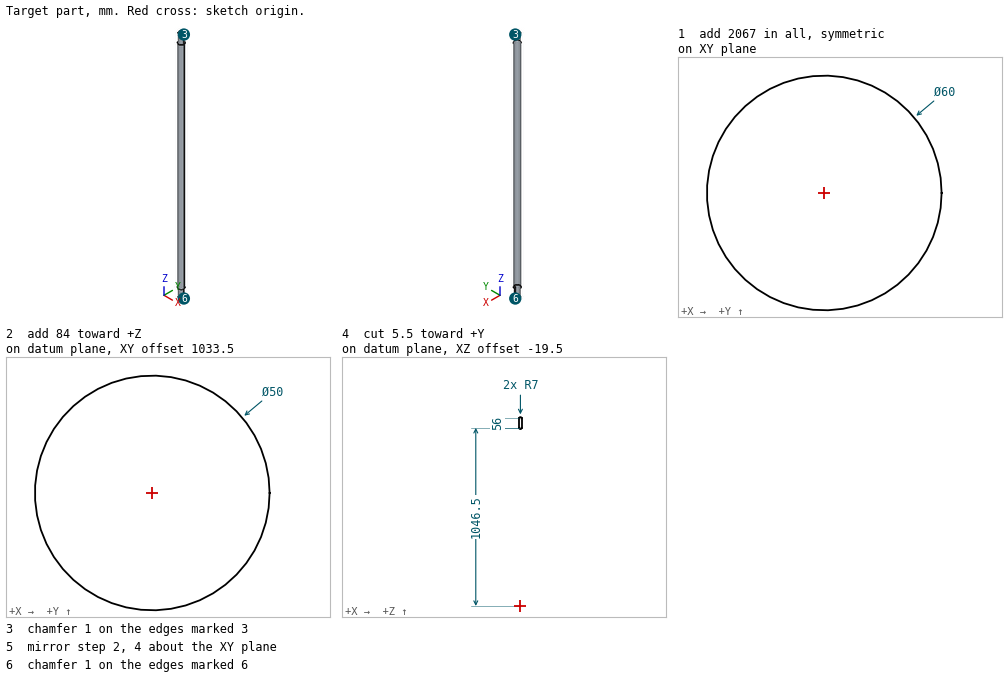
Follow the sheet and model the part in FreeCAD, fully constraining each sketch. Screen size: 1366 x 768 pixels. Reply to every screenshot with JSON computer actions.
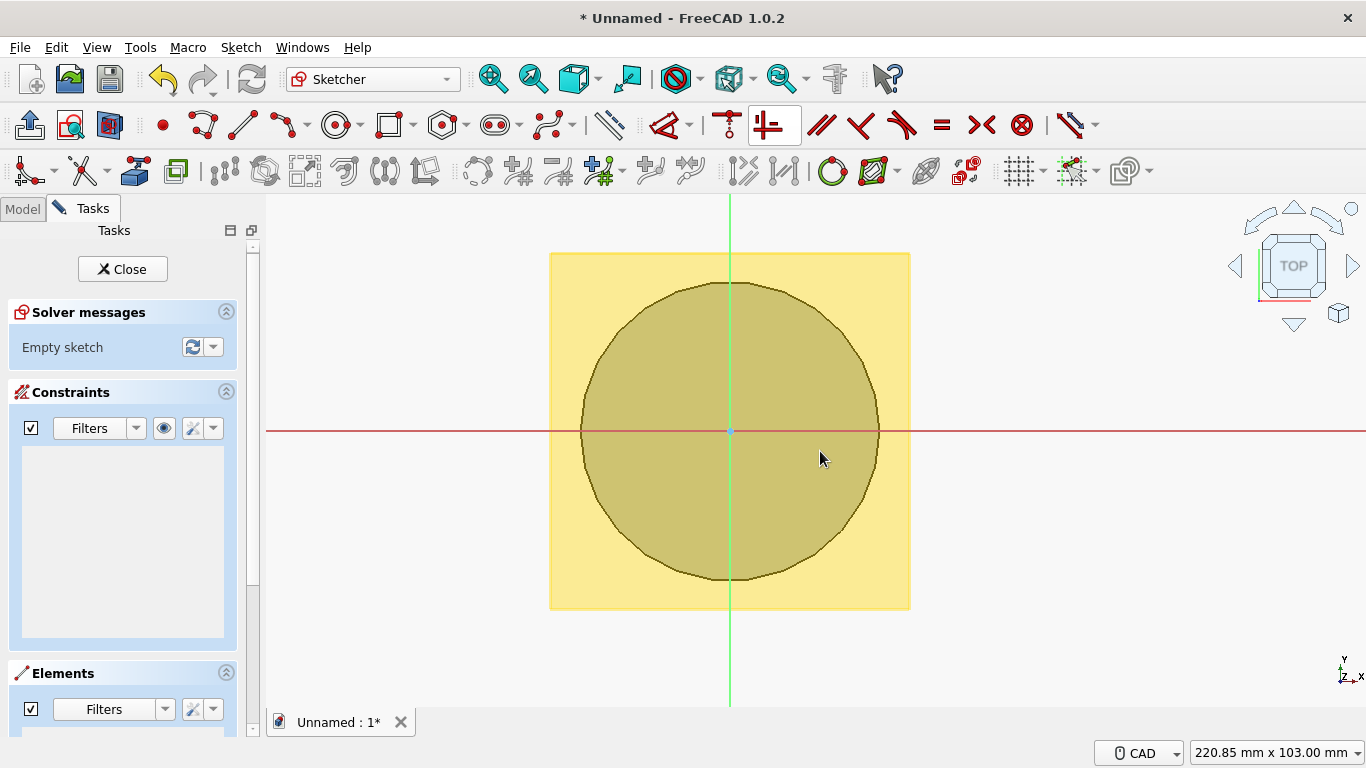
{"action": "left_click", "coordinate": [336, 126]}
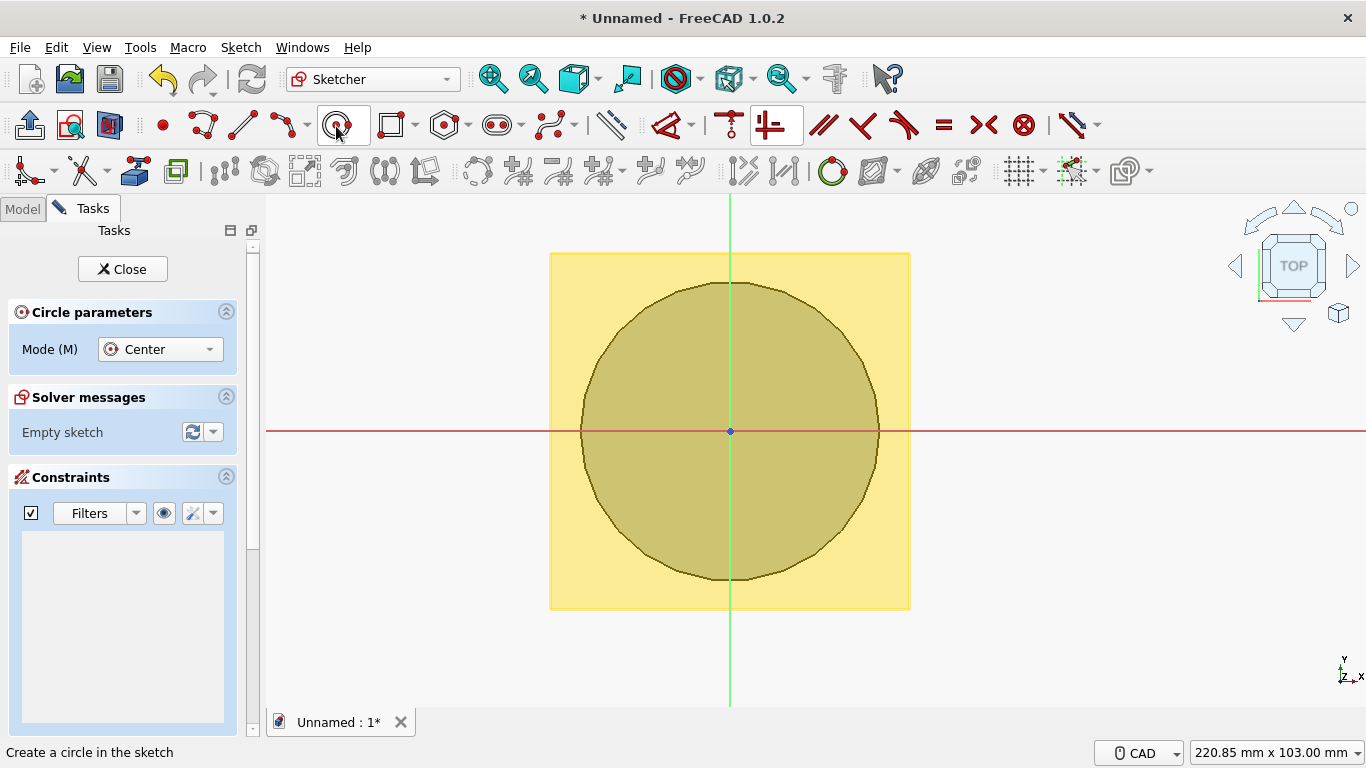
{"action": "left_click", "coordinate": [730, 431]}
{"action": "mouse_move", "coordinate": [818, 343]}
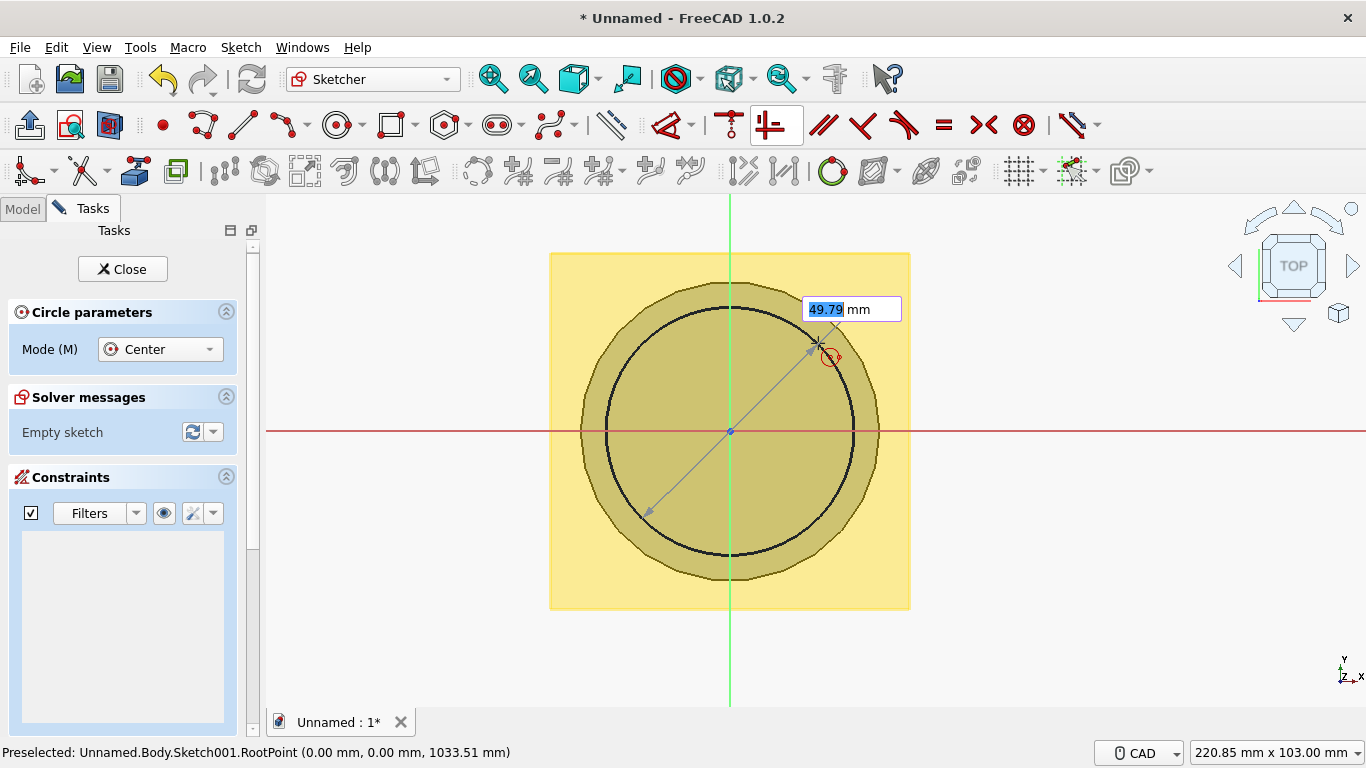
{"action": "type", "text": "50"}
{"action": "key", "text": "Return"}
{"action": "key", "text": "Escape"}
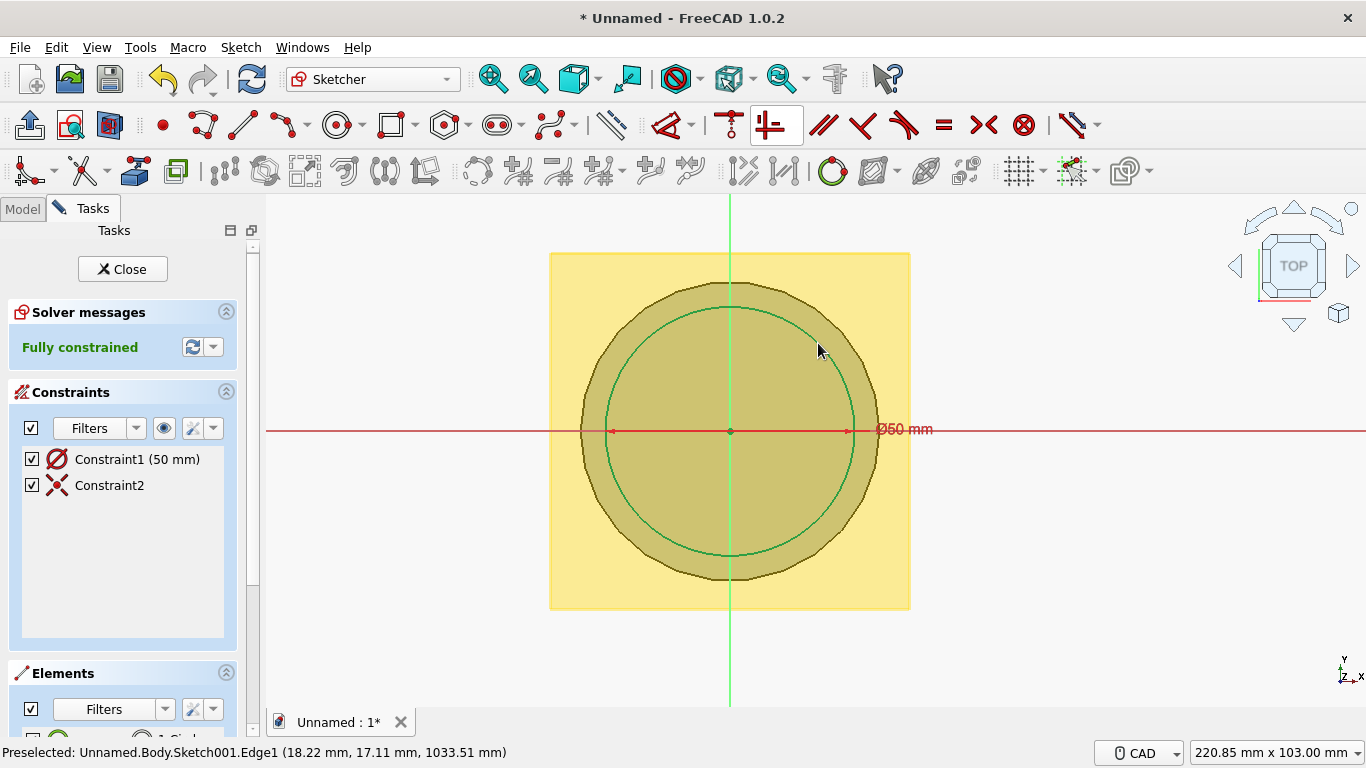
{"action": "left_click", "coordinate": [123, 269]}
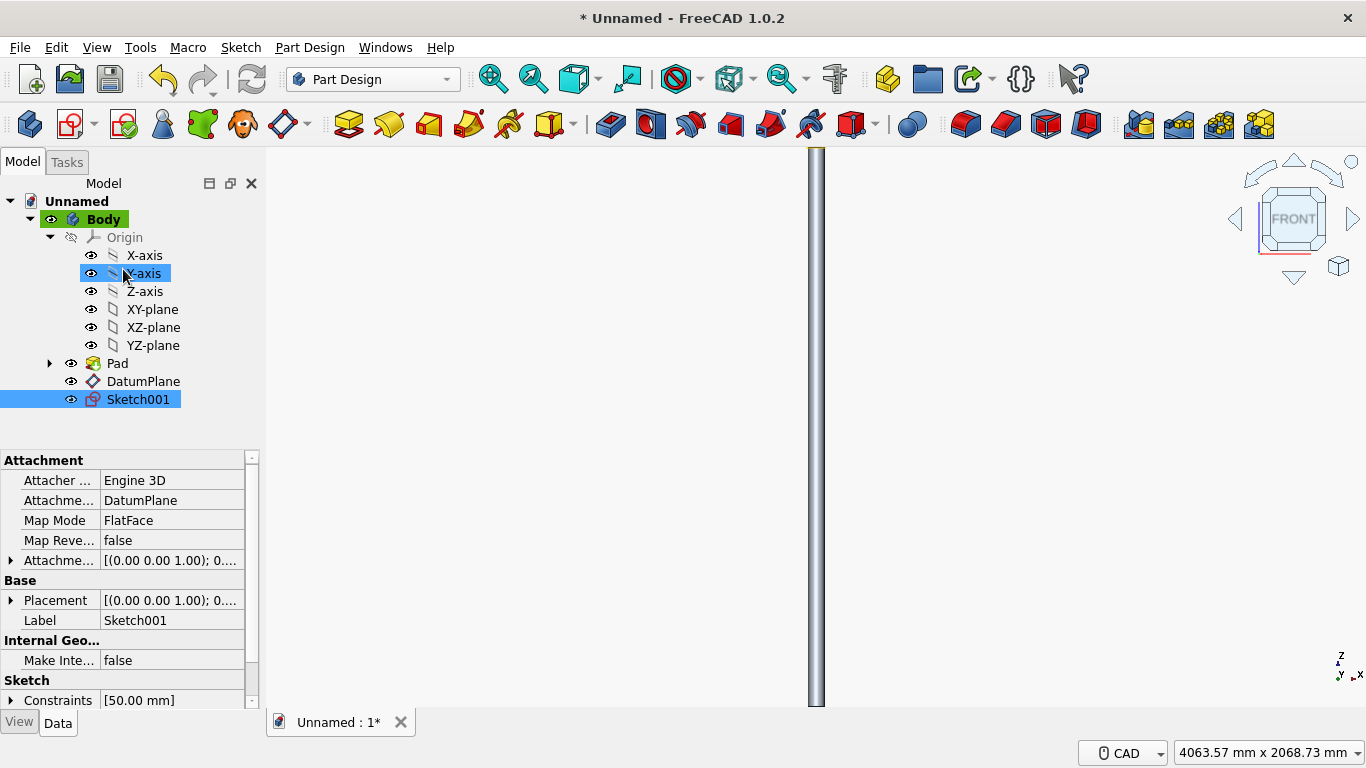
{"action": "left_click", "coordinate": [350, 124]}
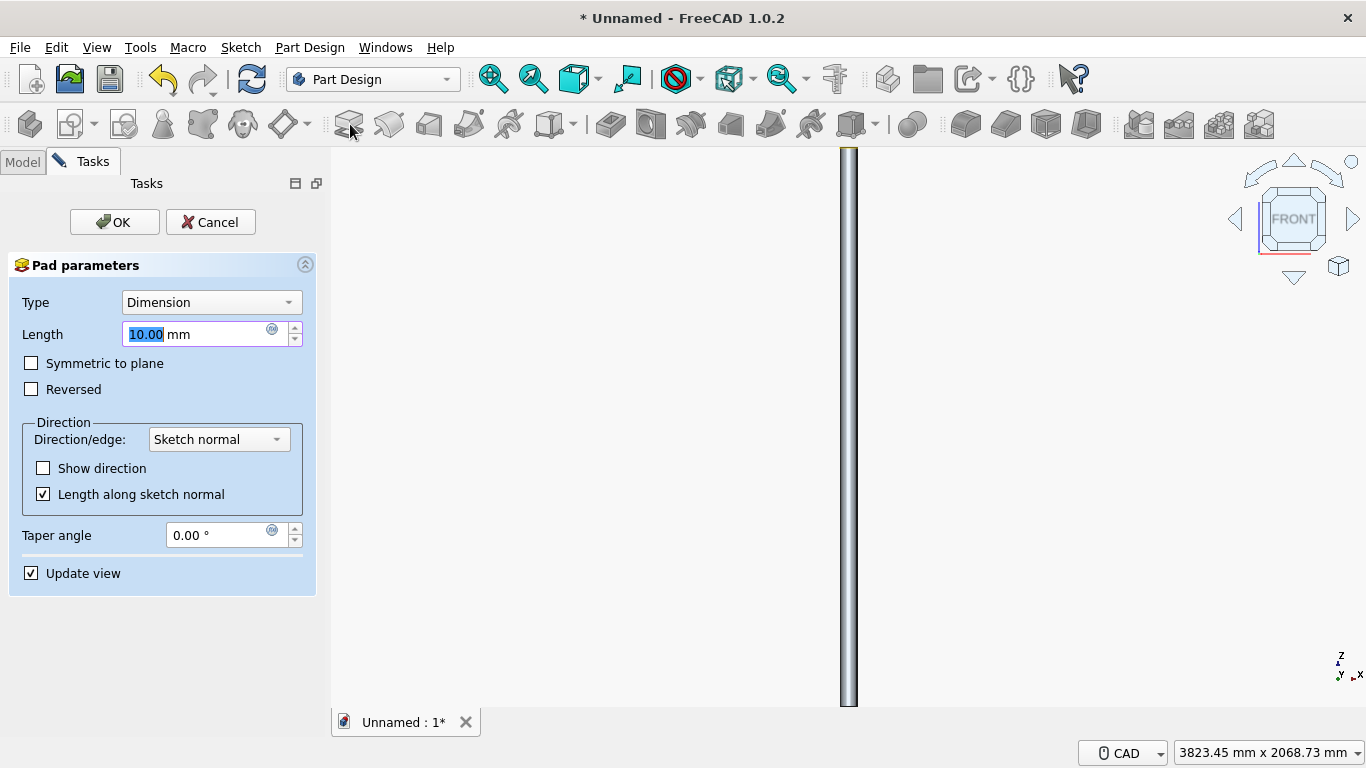
{"action": "type", "text": "84"}
{"action": "key", "text": "Tab"}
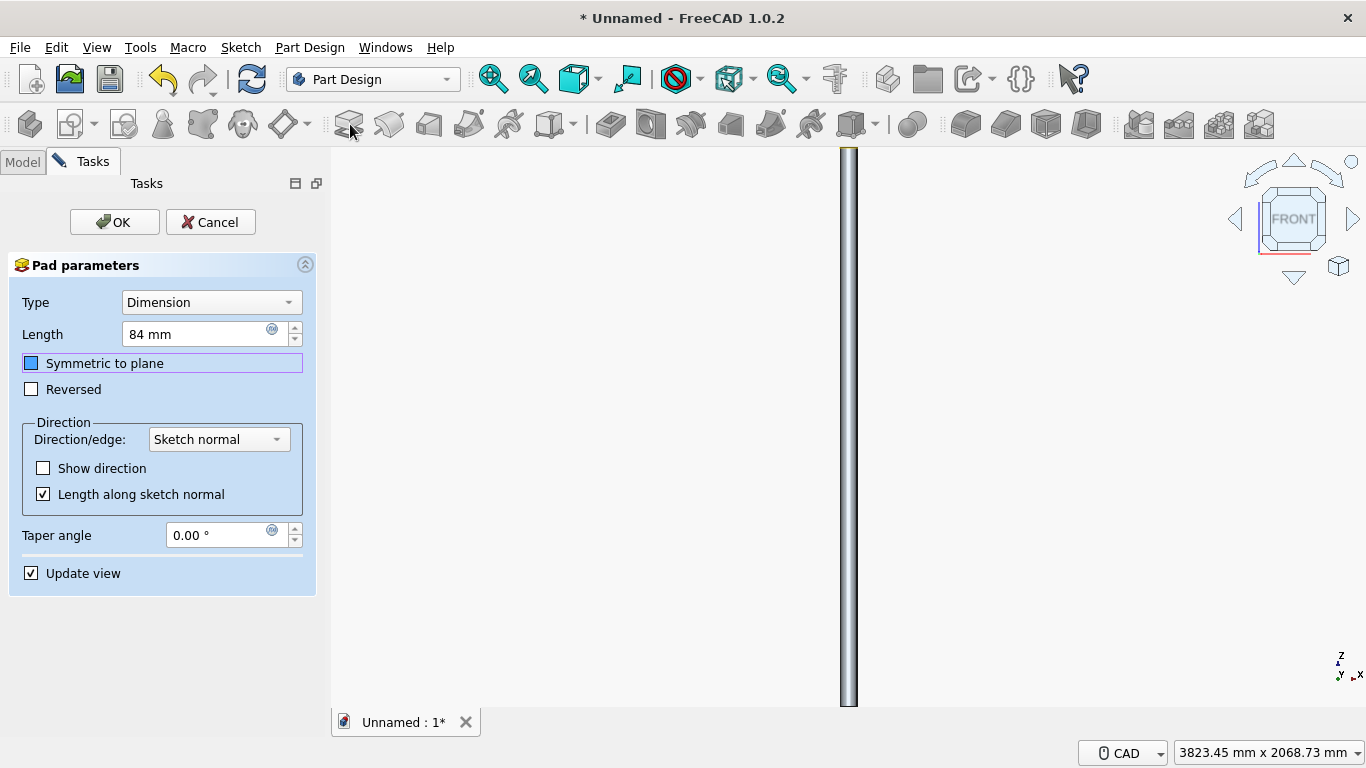
{"action": "left_click", "coordinate": [115, 222]}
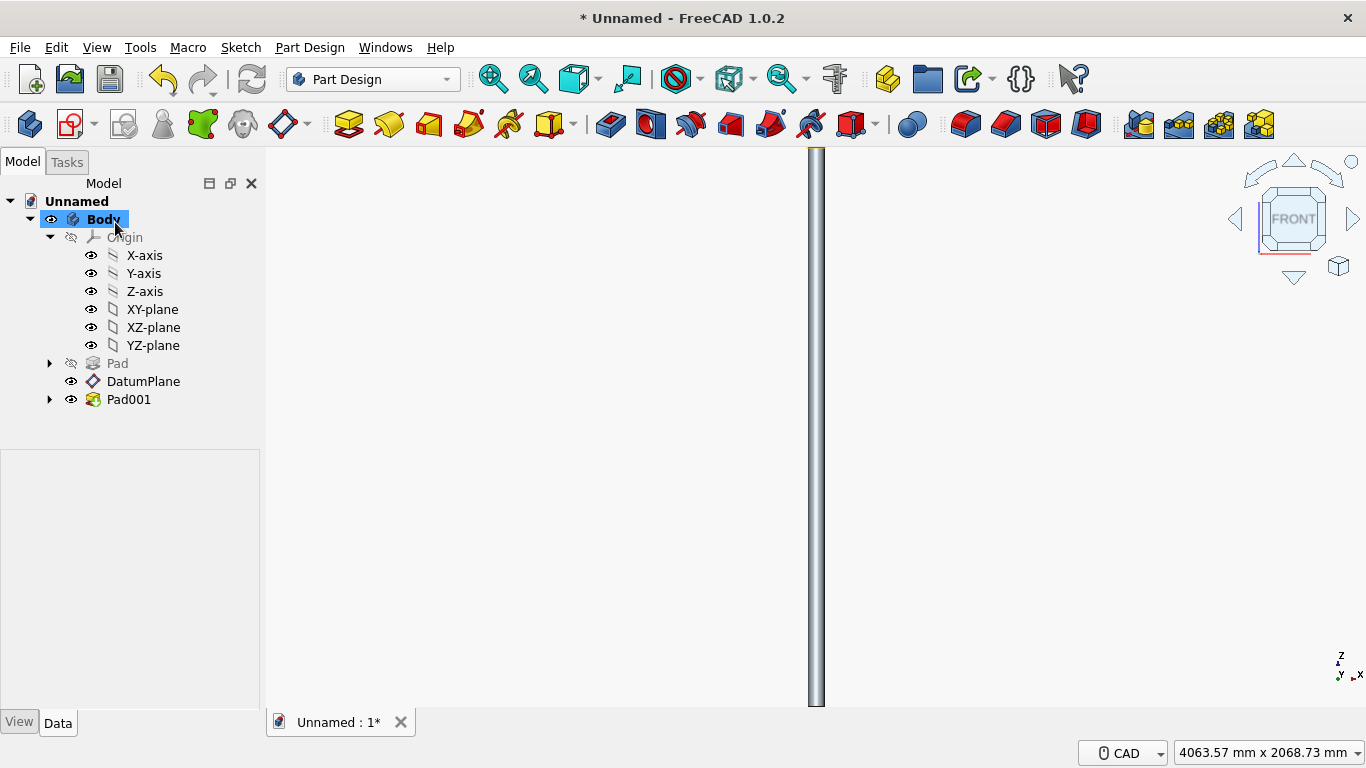
{"action": "left_click", "coordinate": [116, 381]}
{"action": "key", "text": "space"}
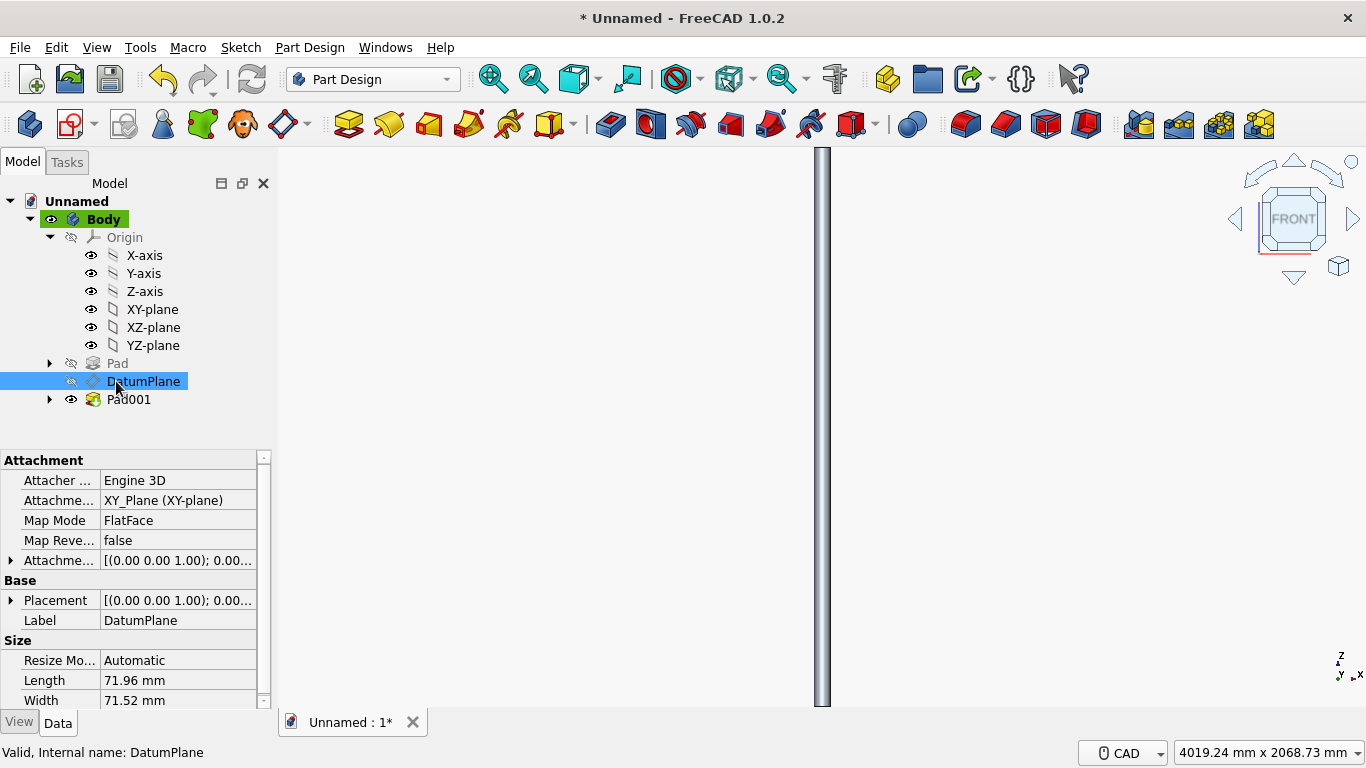
{"action": "left_click", "coordinate": [494, 80]}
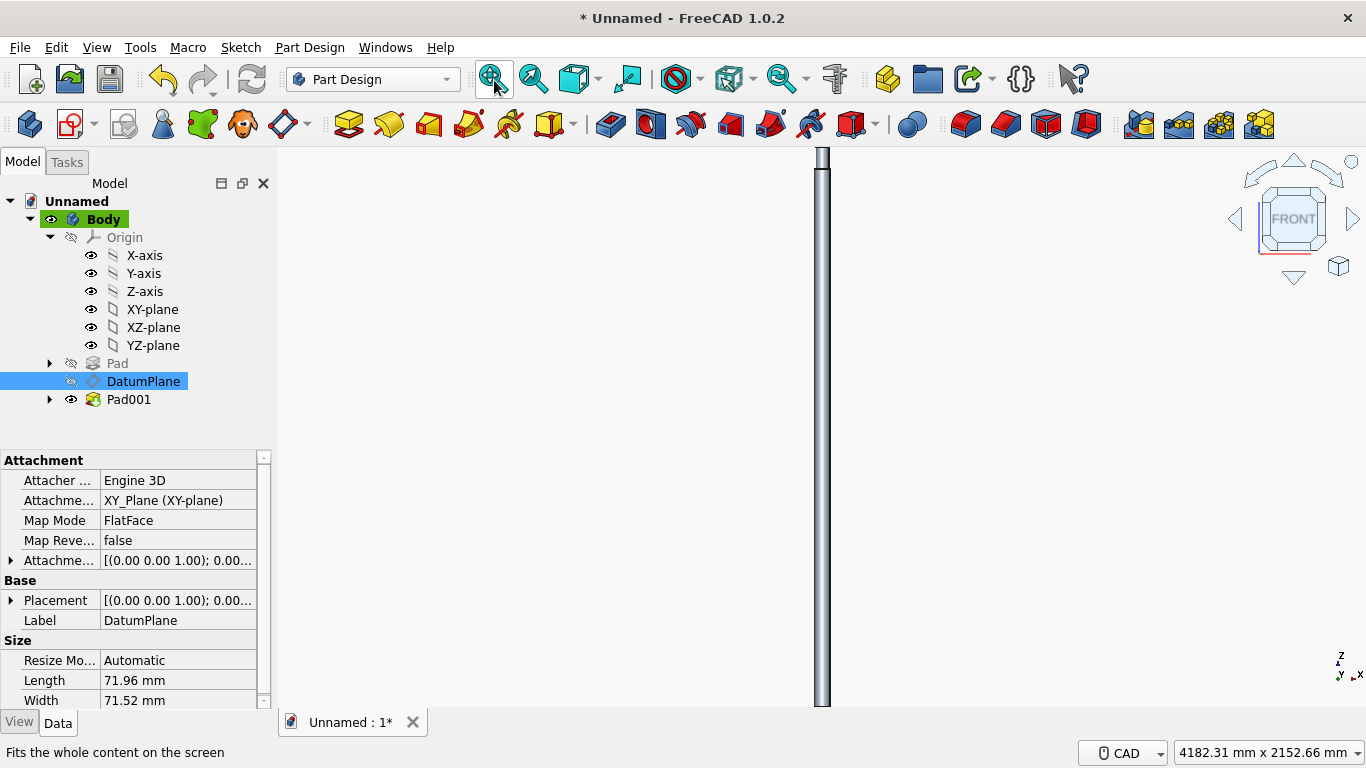
{"action": "key", "text": "0"}